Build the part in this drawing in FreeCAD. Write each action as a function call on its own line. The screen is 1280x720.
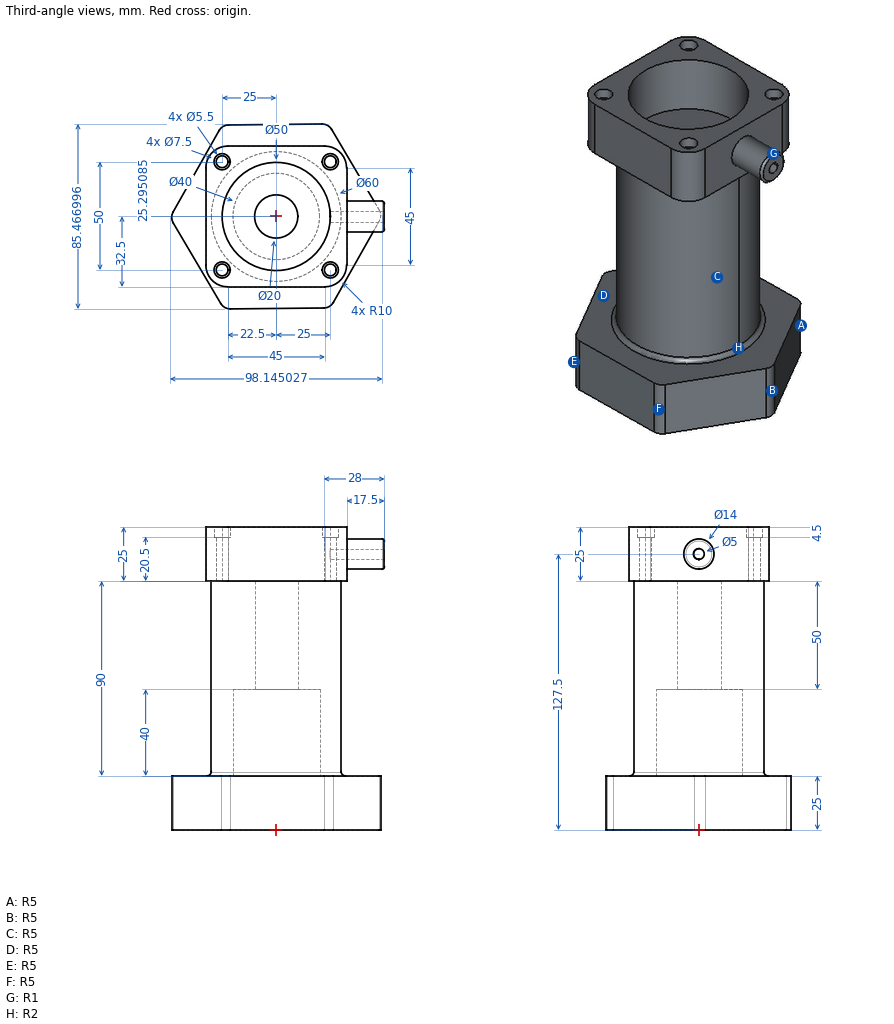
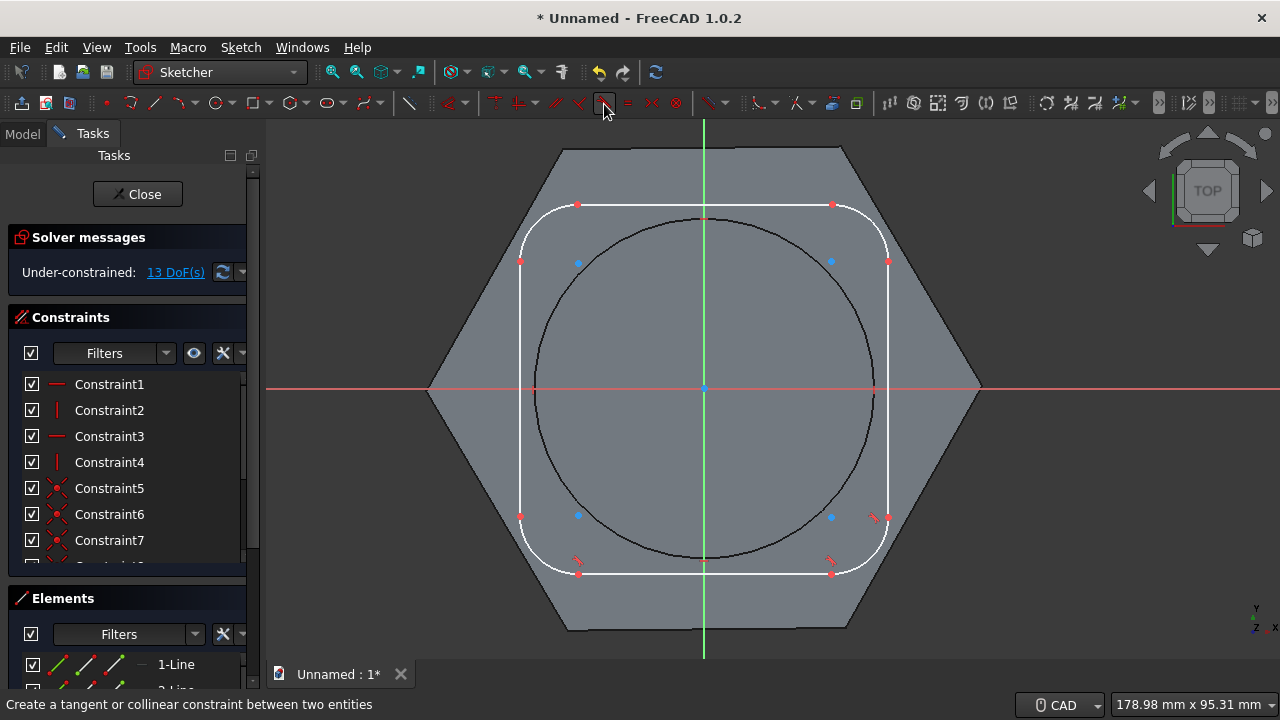
click(888, 441)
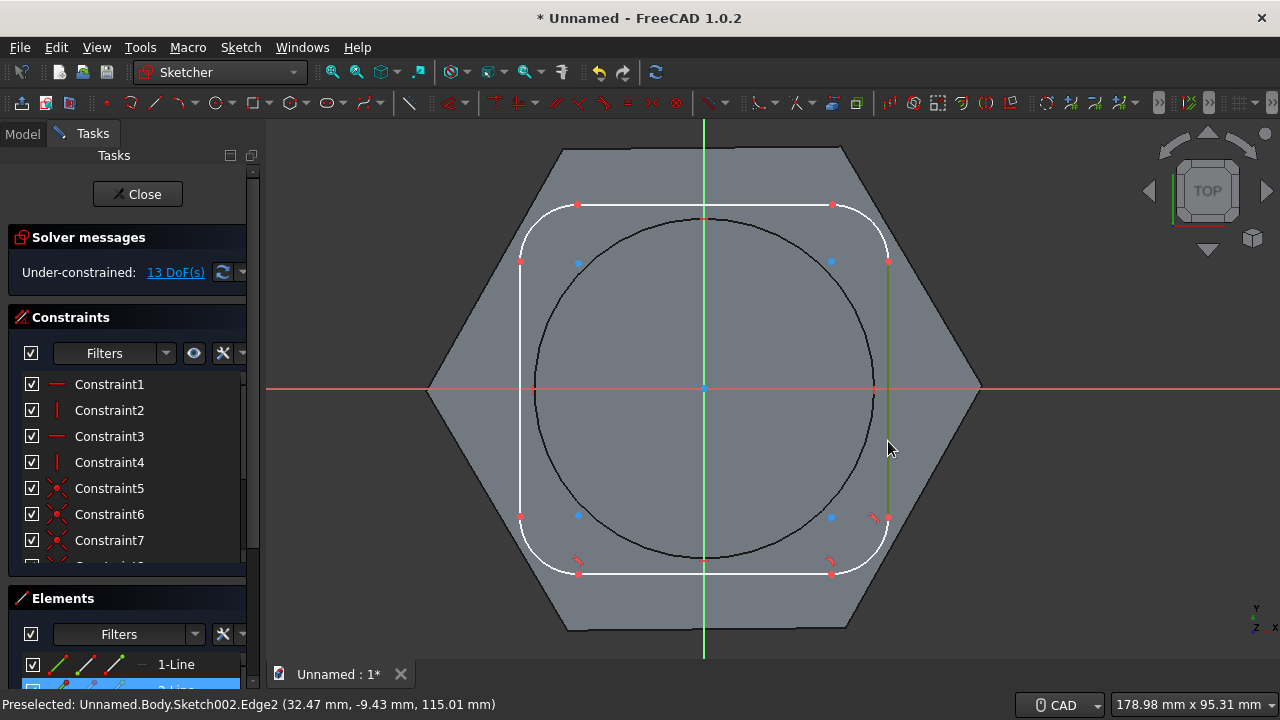
click(882, 236)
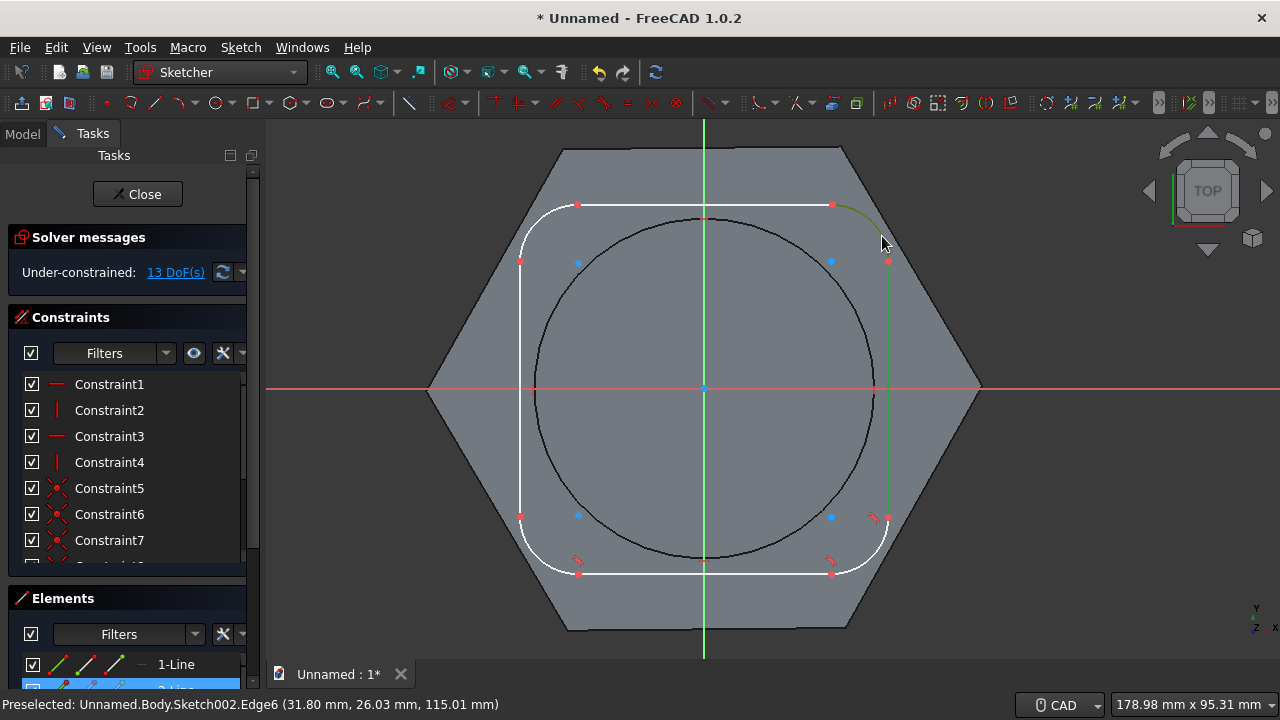
click(604, 104)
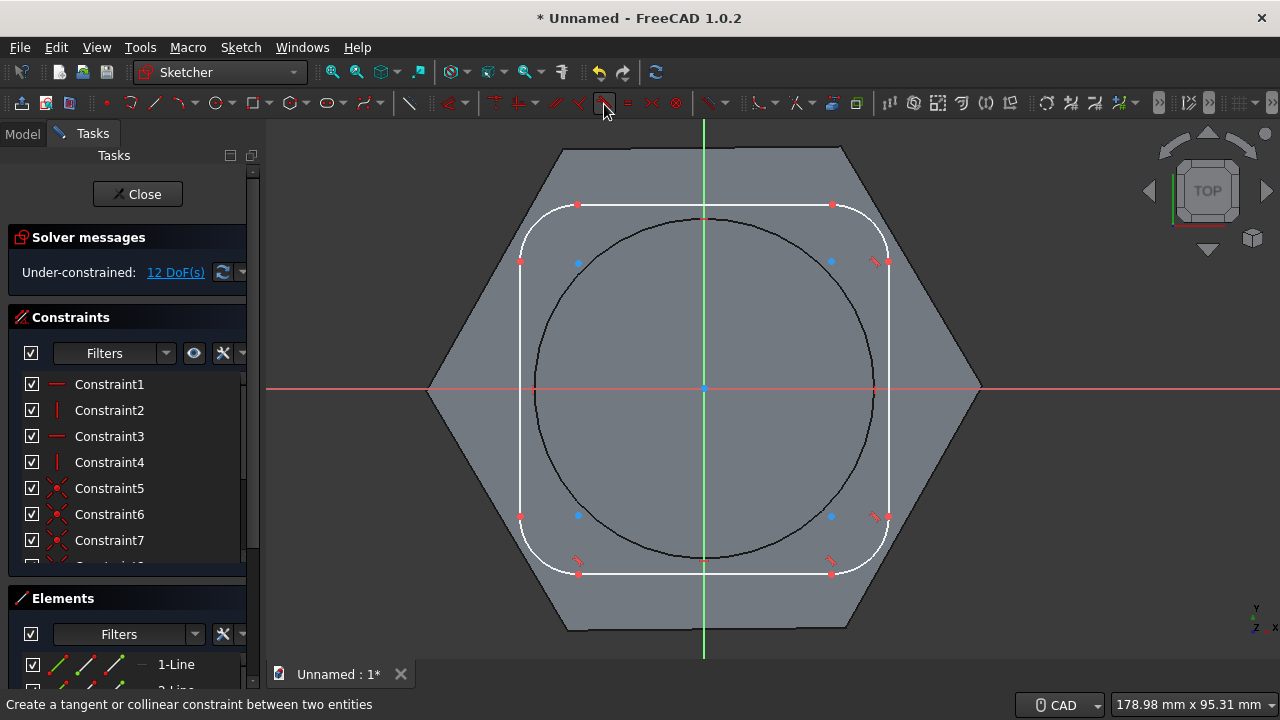
click(755, 205)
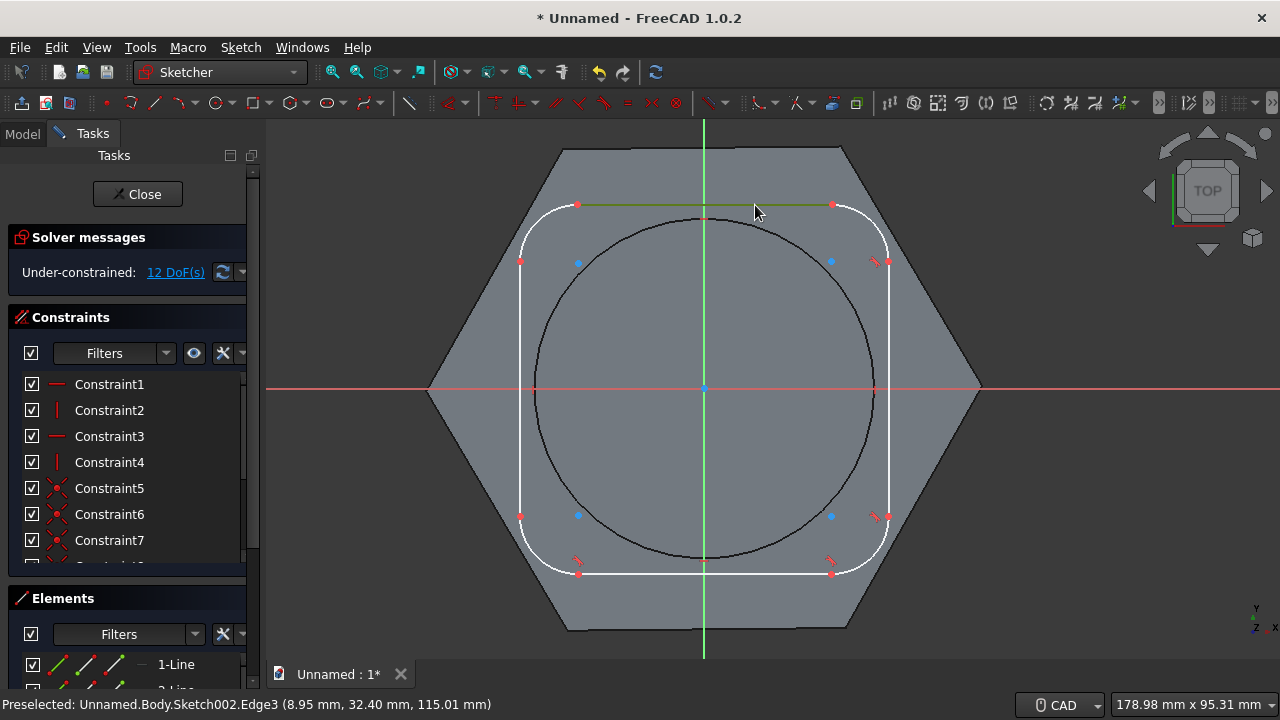
click(883, 236)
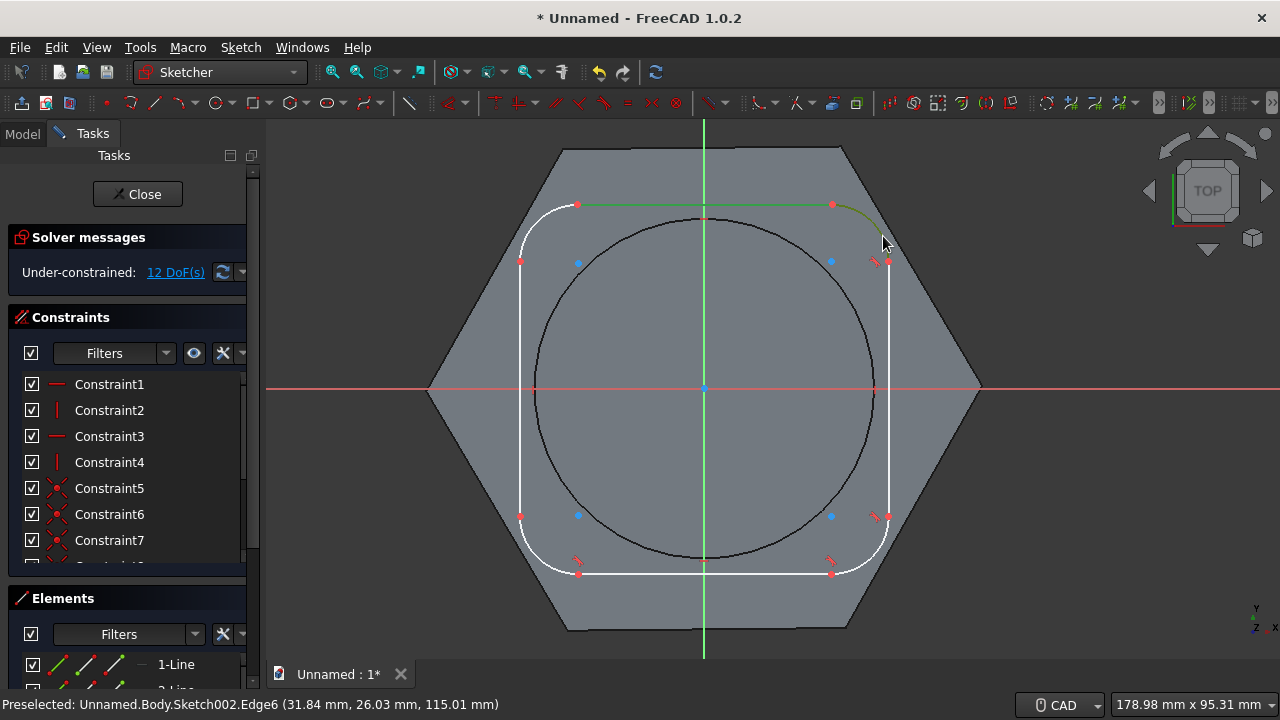
click(604, 104)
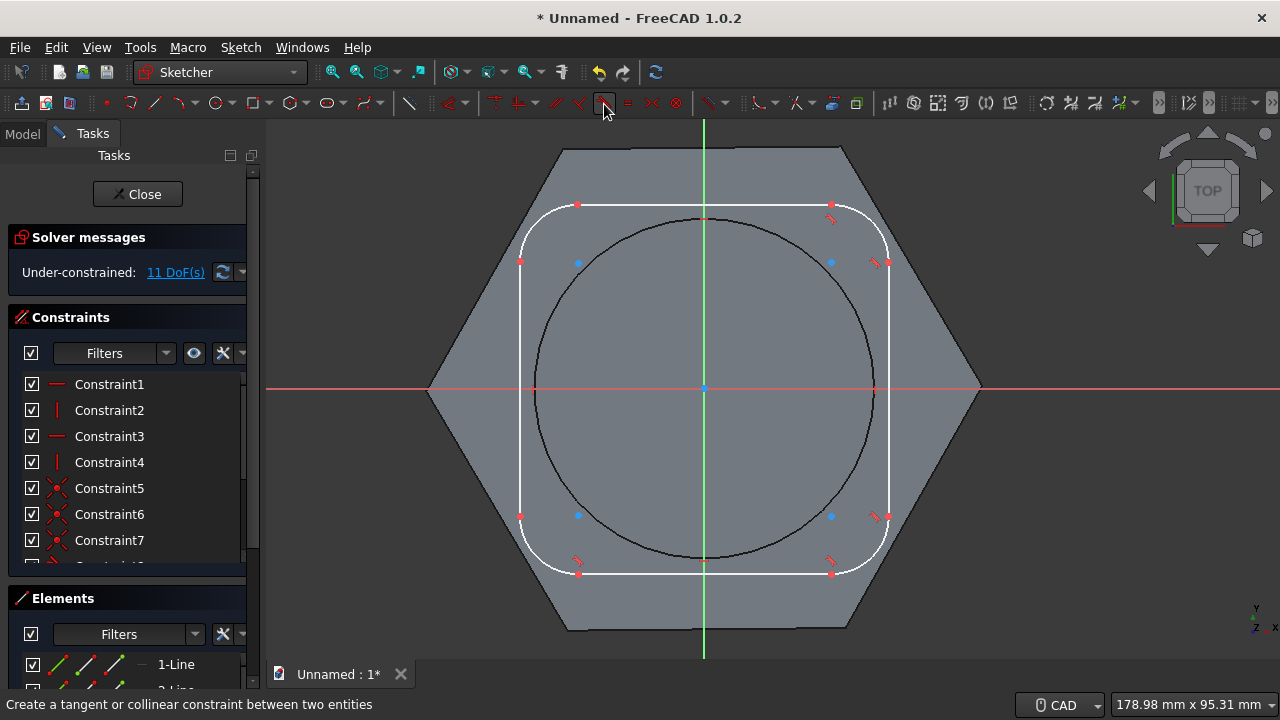
click(755, 205)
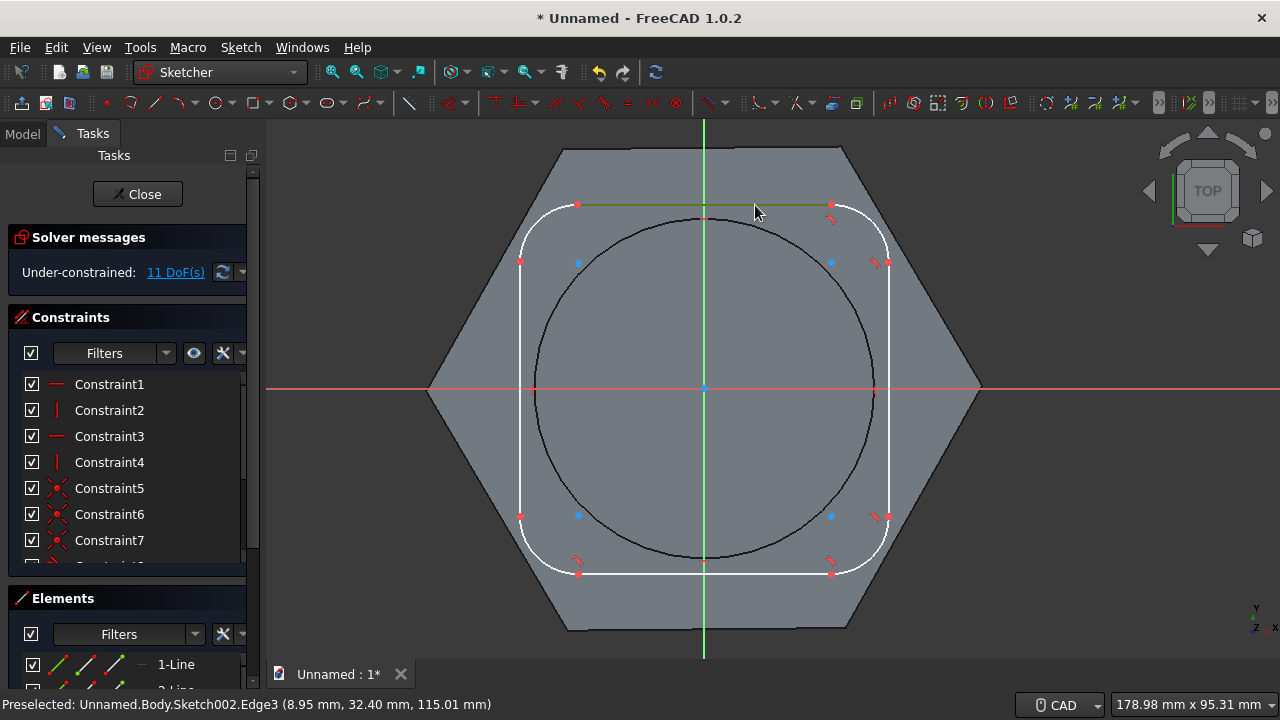
click(551, 212)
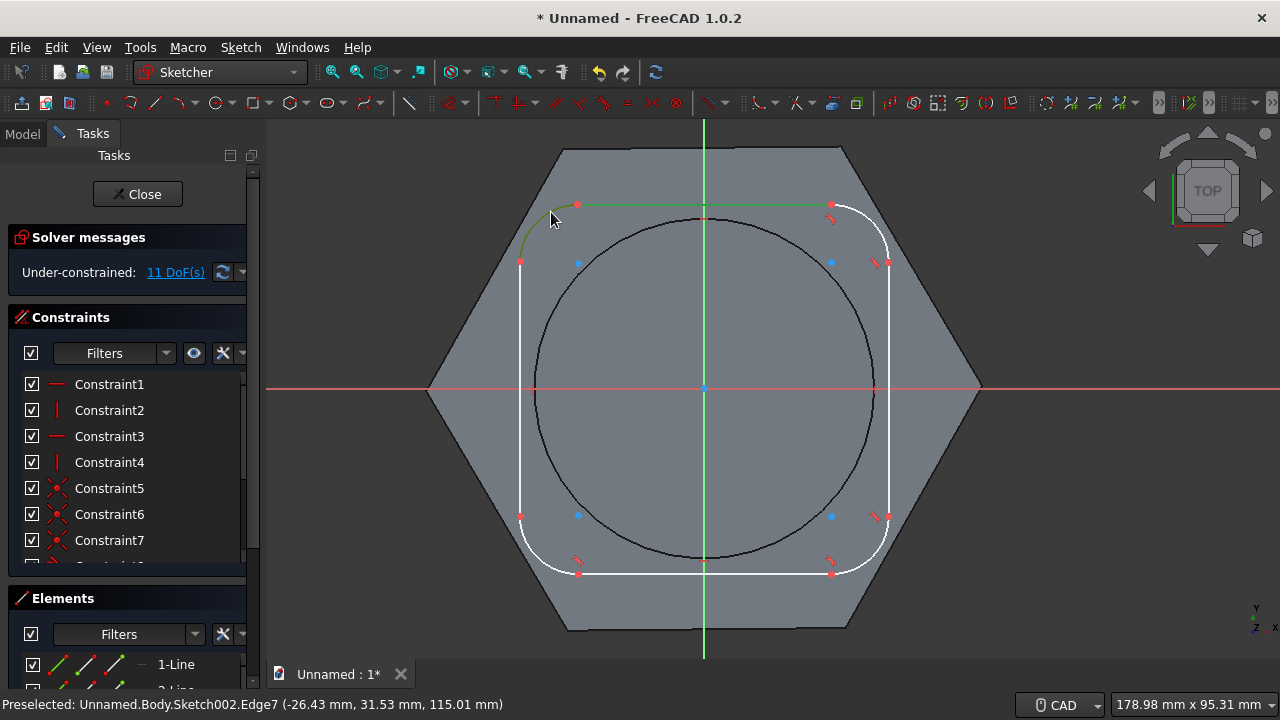
key(t)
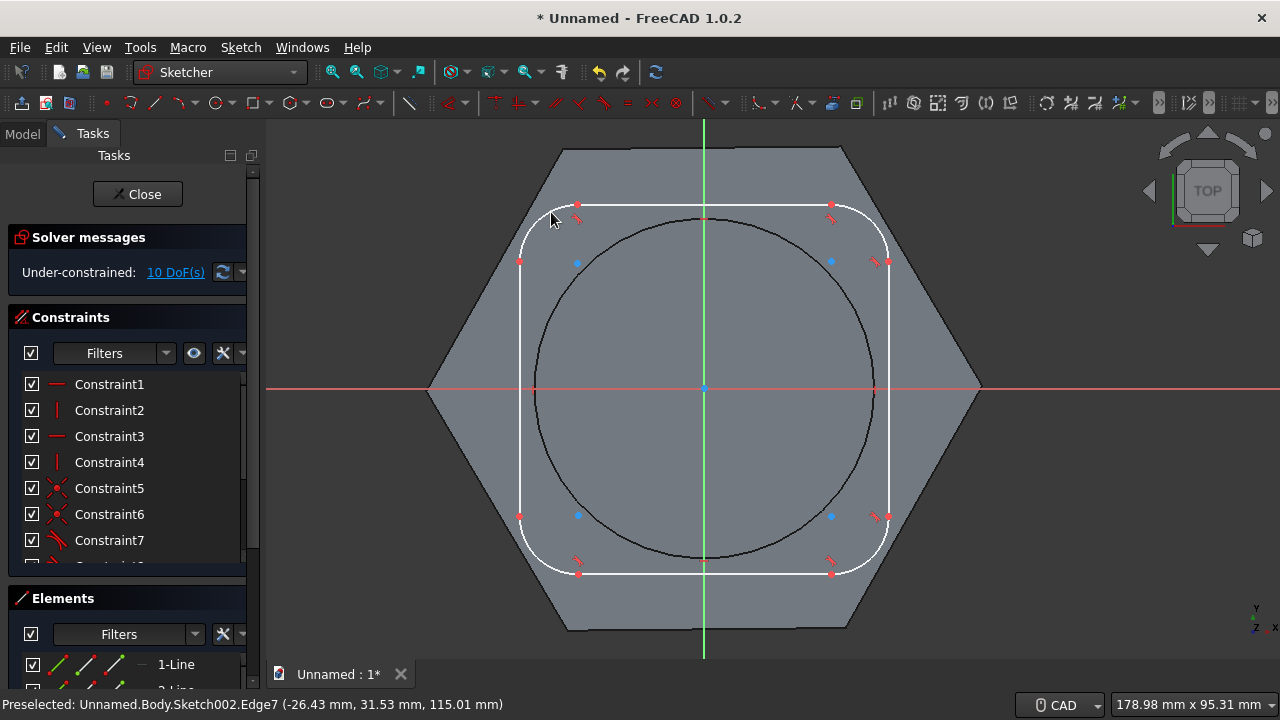
click(520, 338)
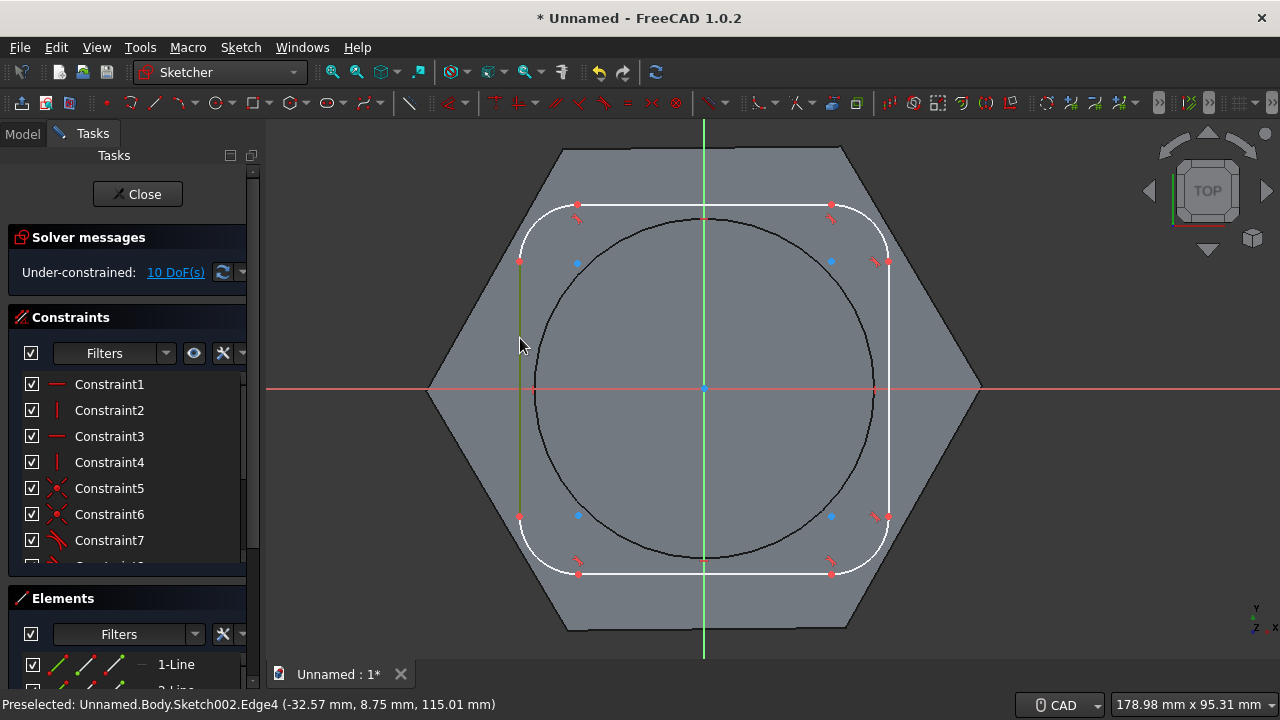
click(552, 211)